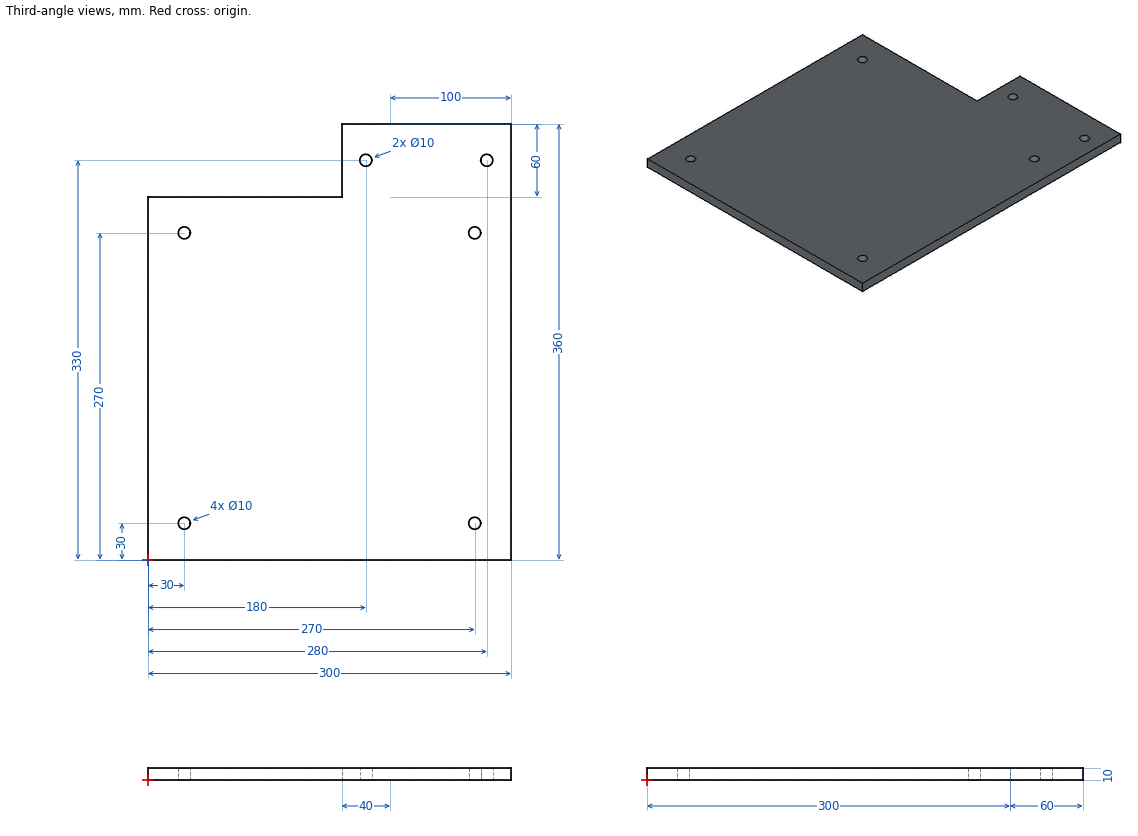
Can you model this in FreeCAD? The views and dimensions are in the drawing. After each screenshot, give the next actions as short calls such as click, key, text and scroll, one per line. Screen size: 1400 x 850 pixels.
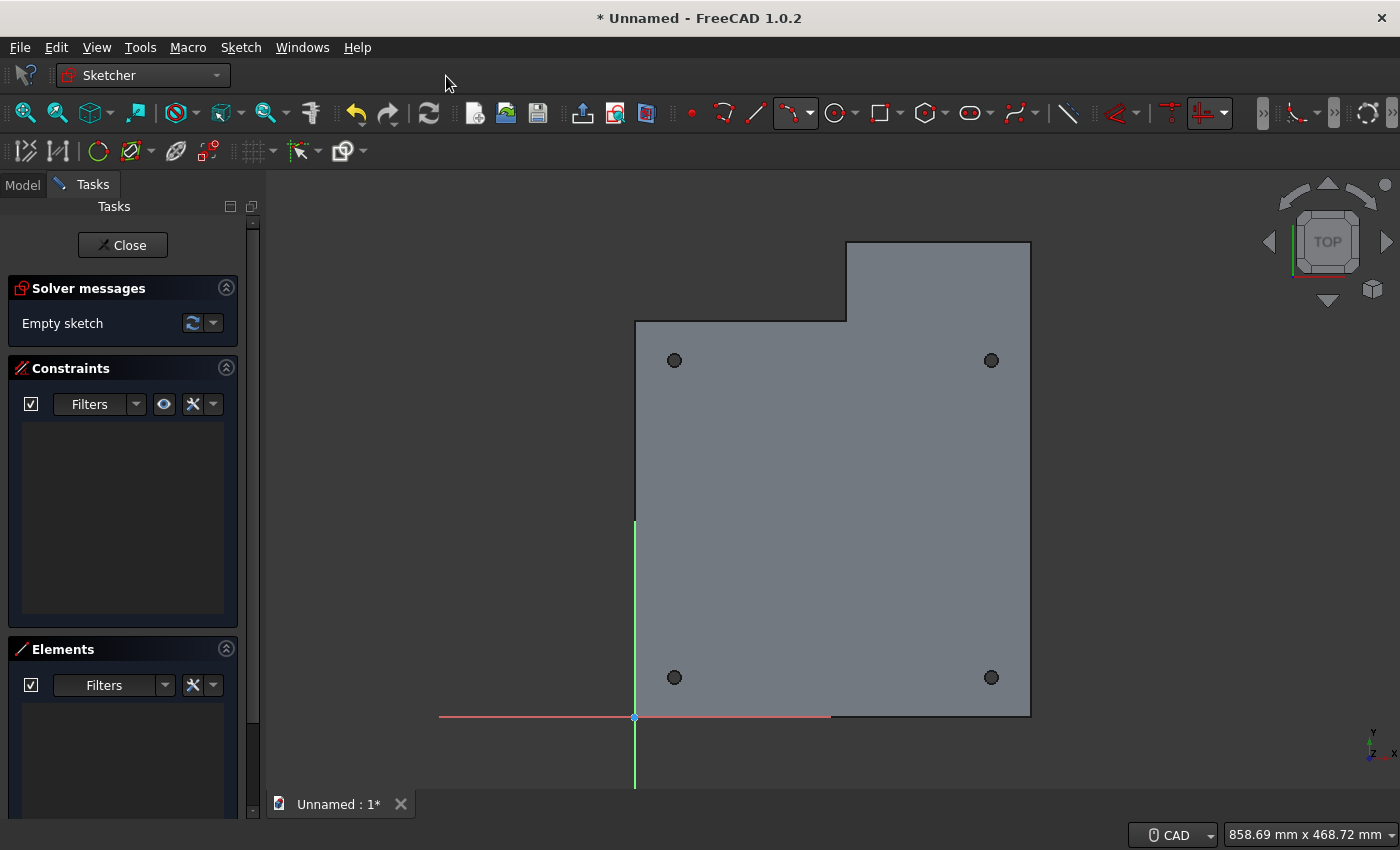
scroll(983, 231, up, 8)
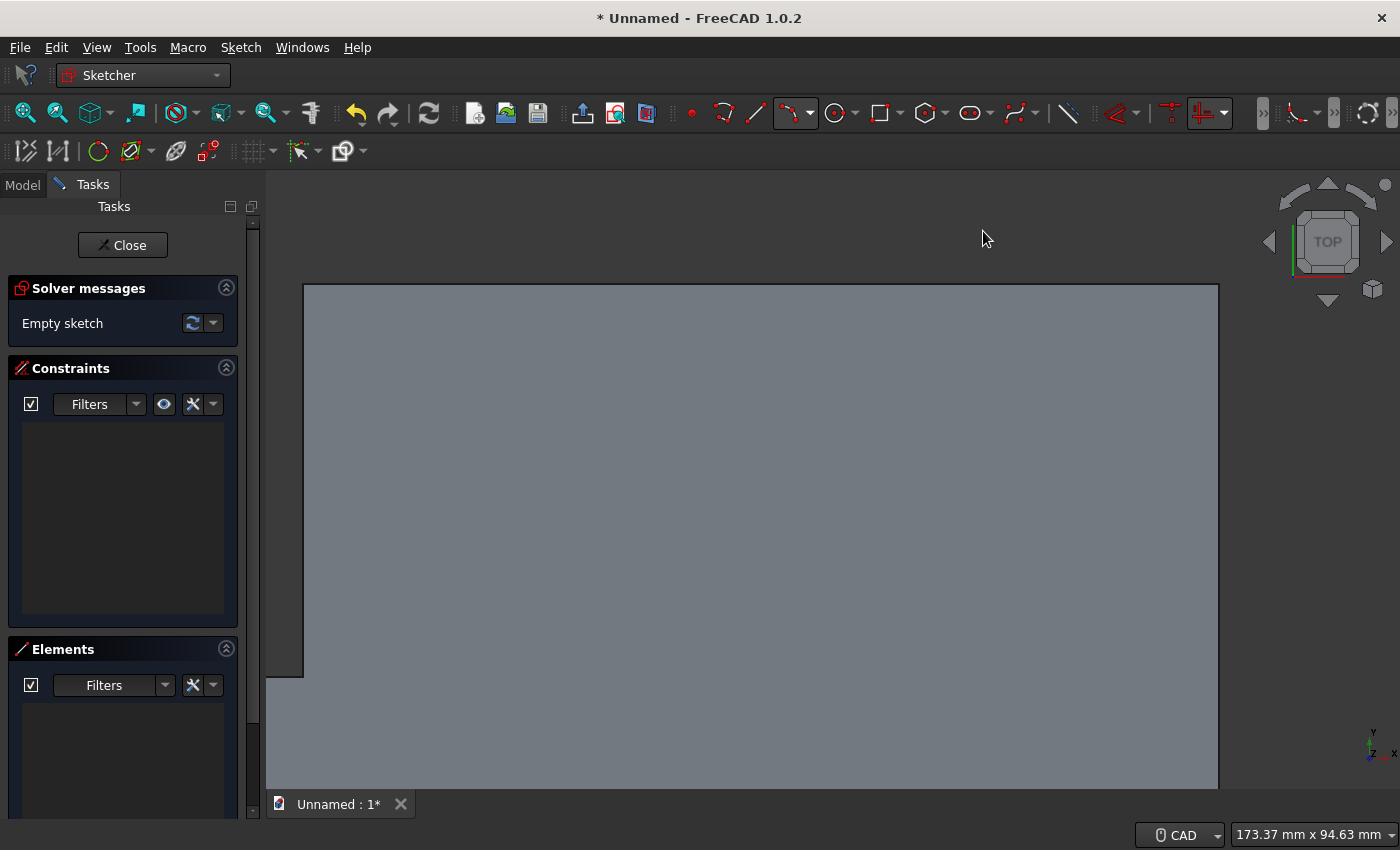
click(836, 114)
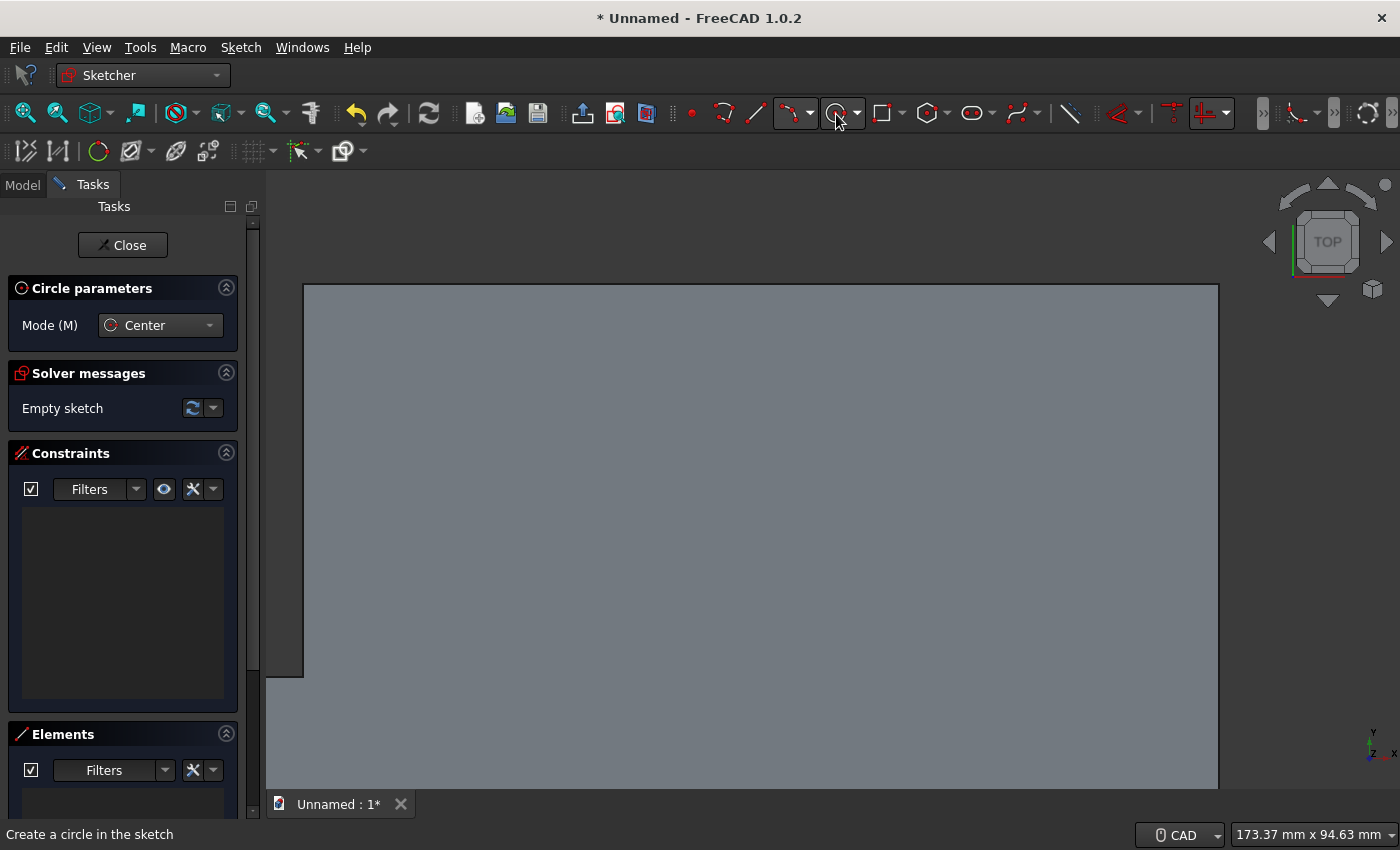
click(434, 480)
move(457, 457)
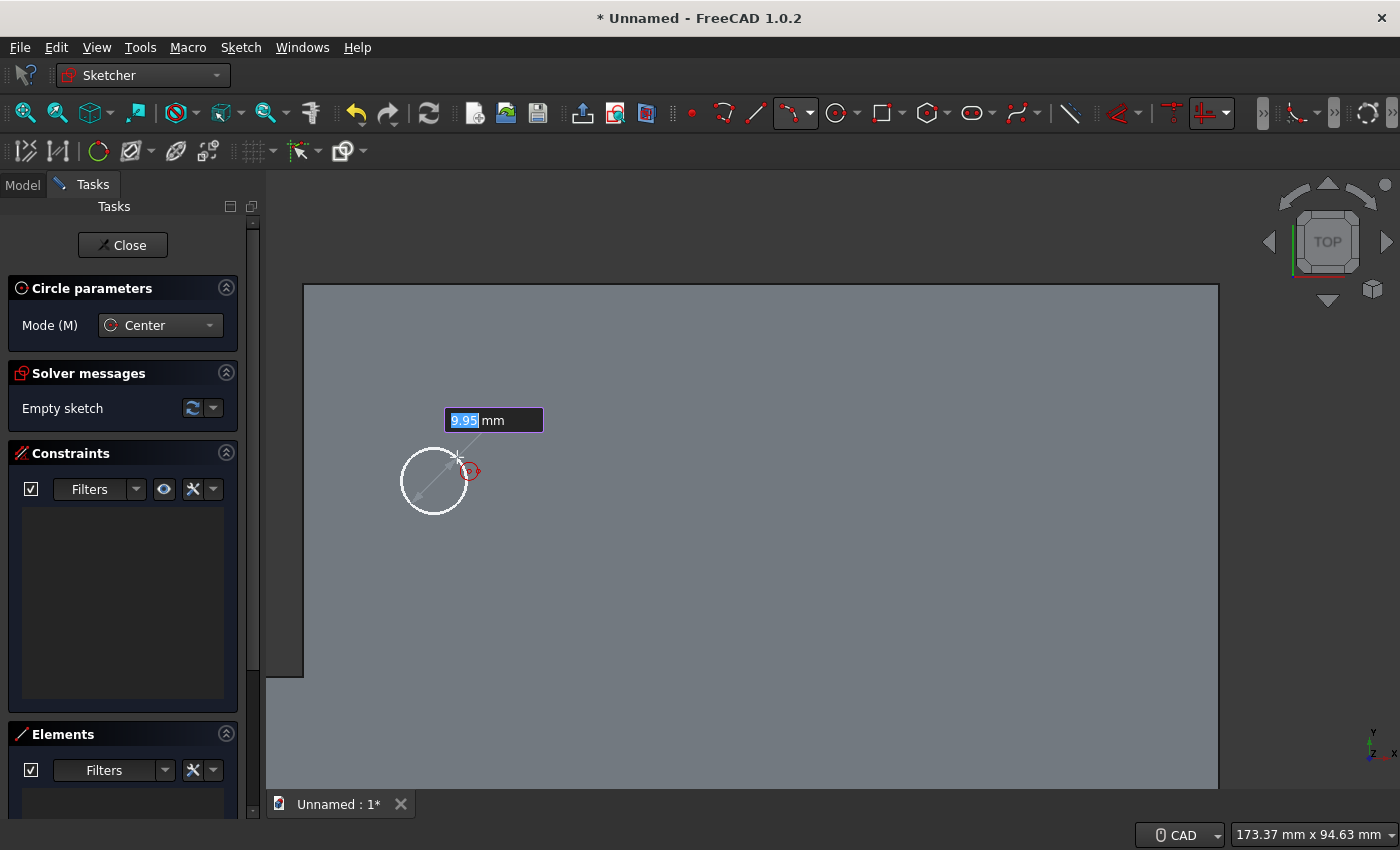
text(10)
key(Return)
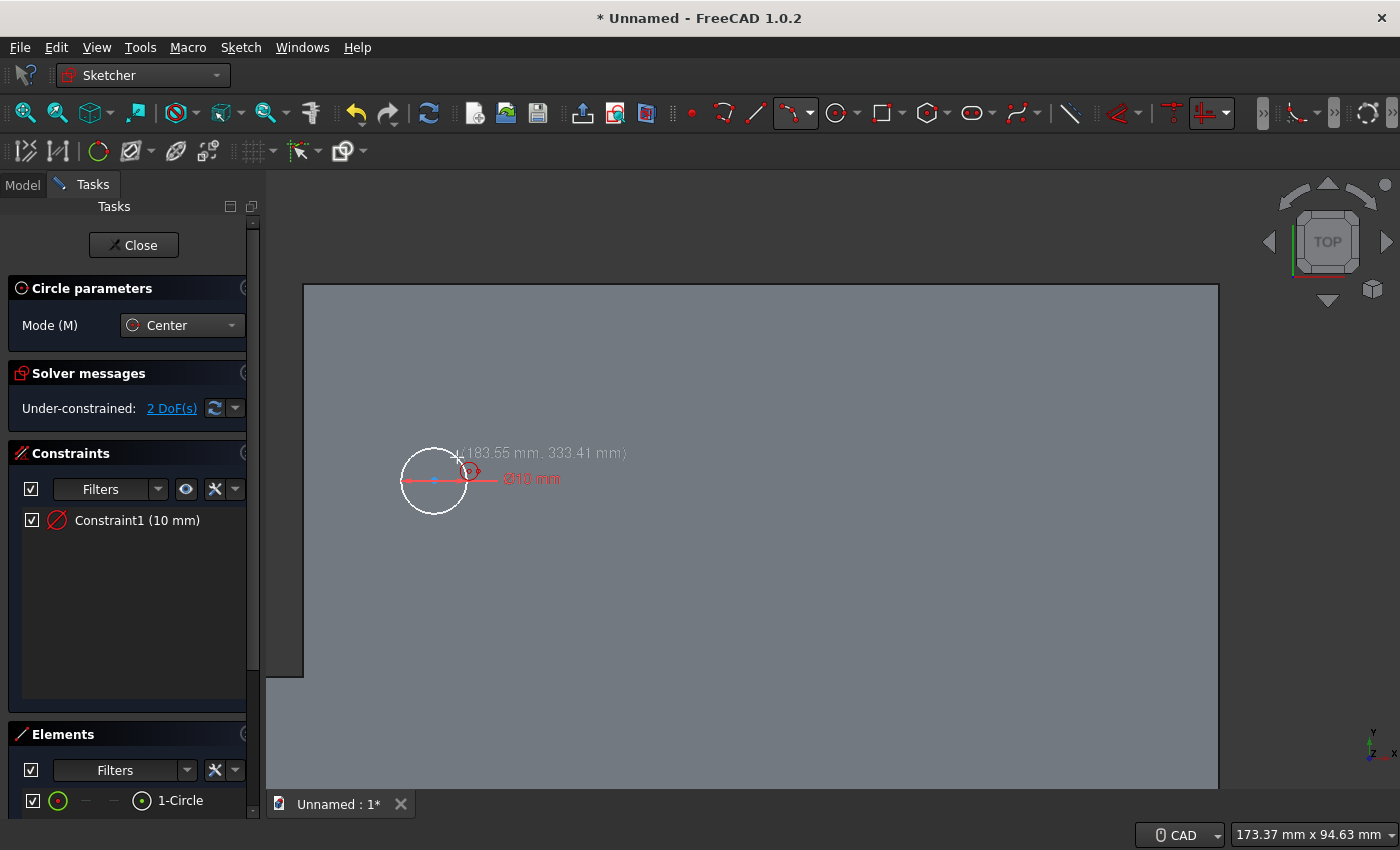
click(1088, 480)
move(1111, 457)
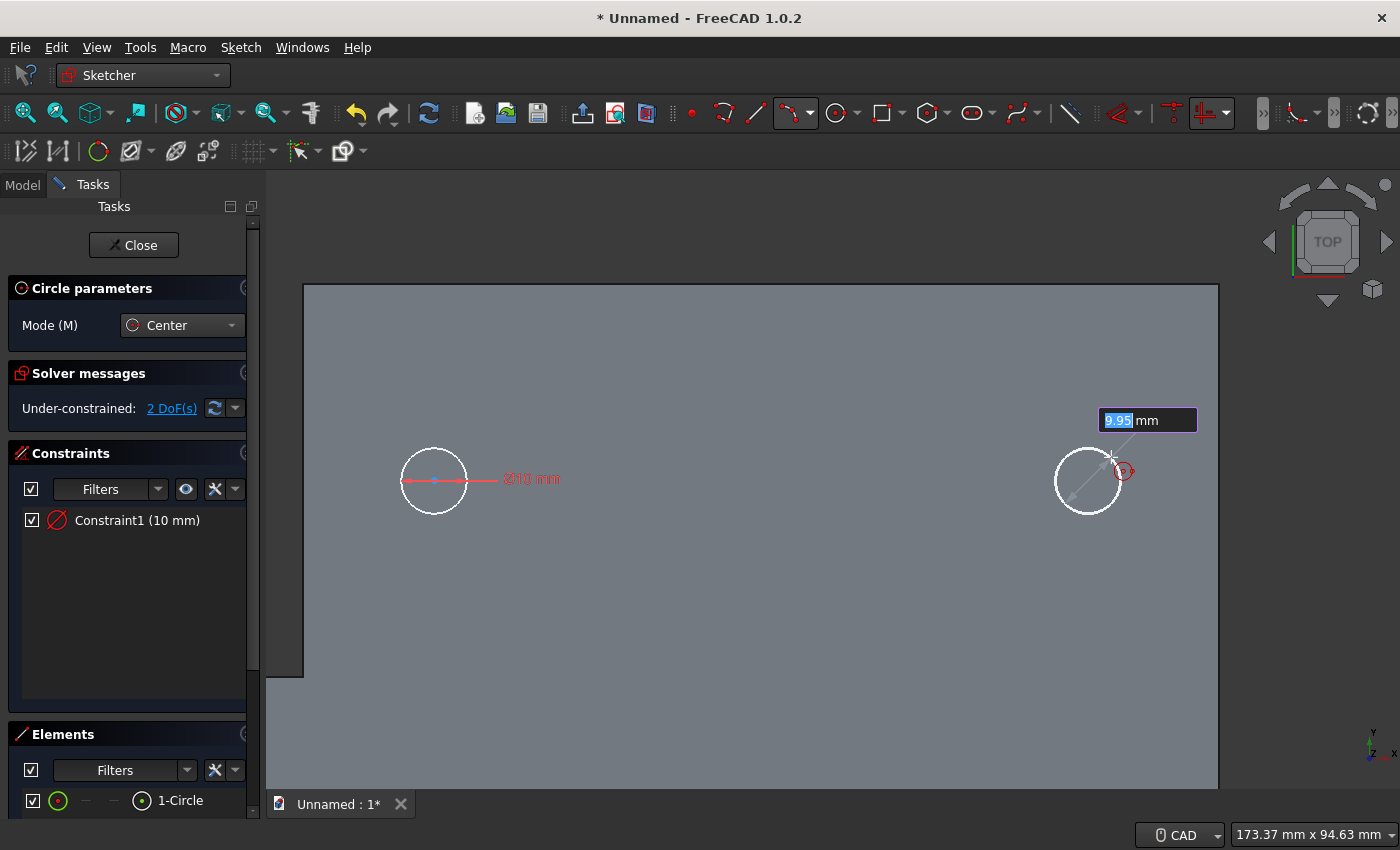
text(10)
key(Return)
key(Escape)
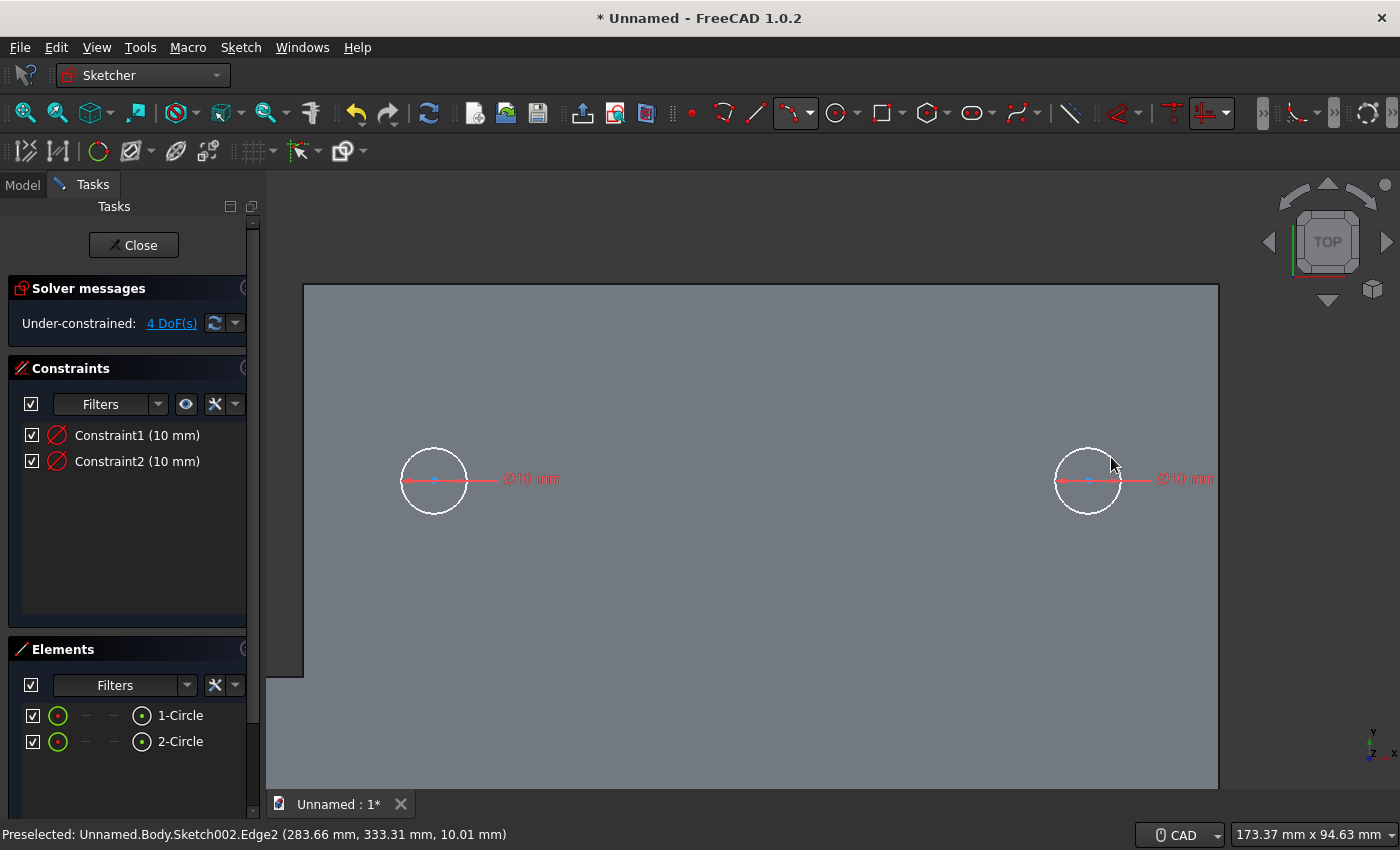
click(434, 481)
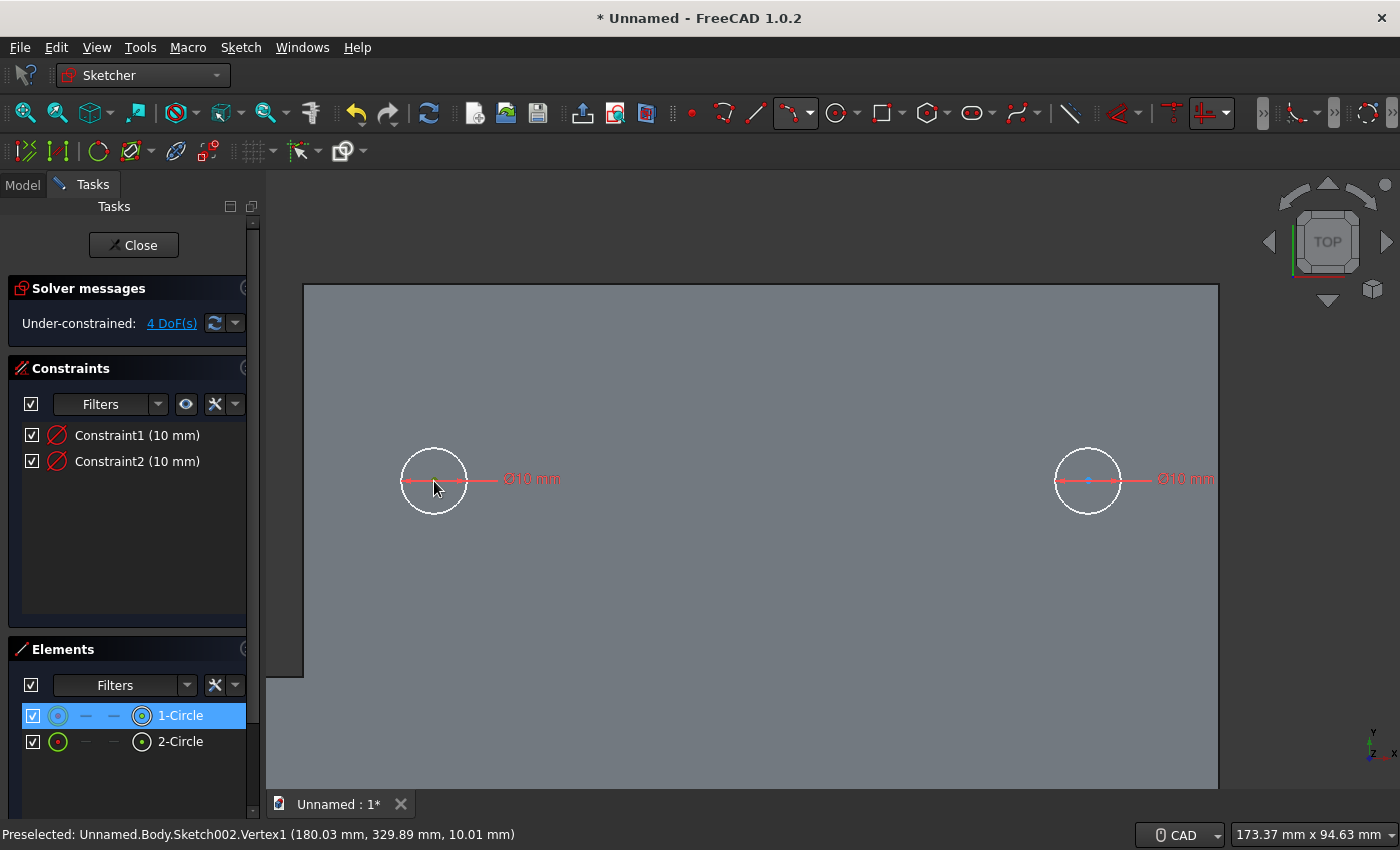
click(1088, 481)